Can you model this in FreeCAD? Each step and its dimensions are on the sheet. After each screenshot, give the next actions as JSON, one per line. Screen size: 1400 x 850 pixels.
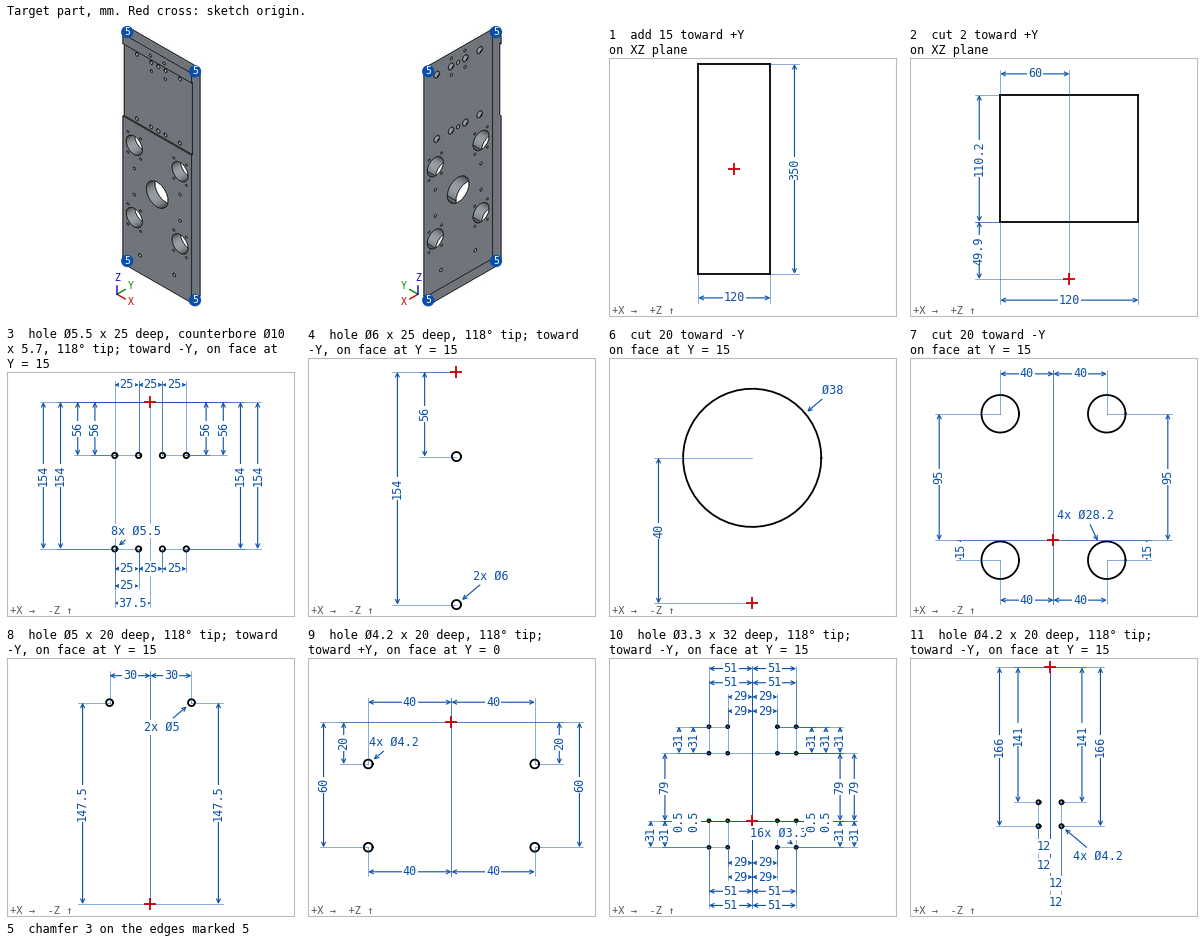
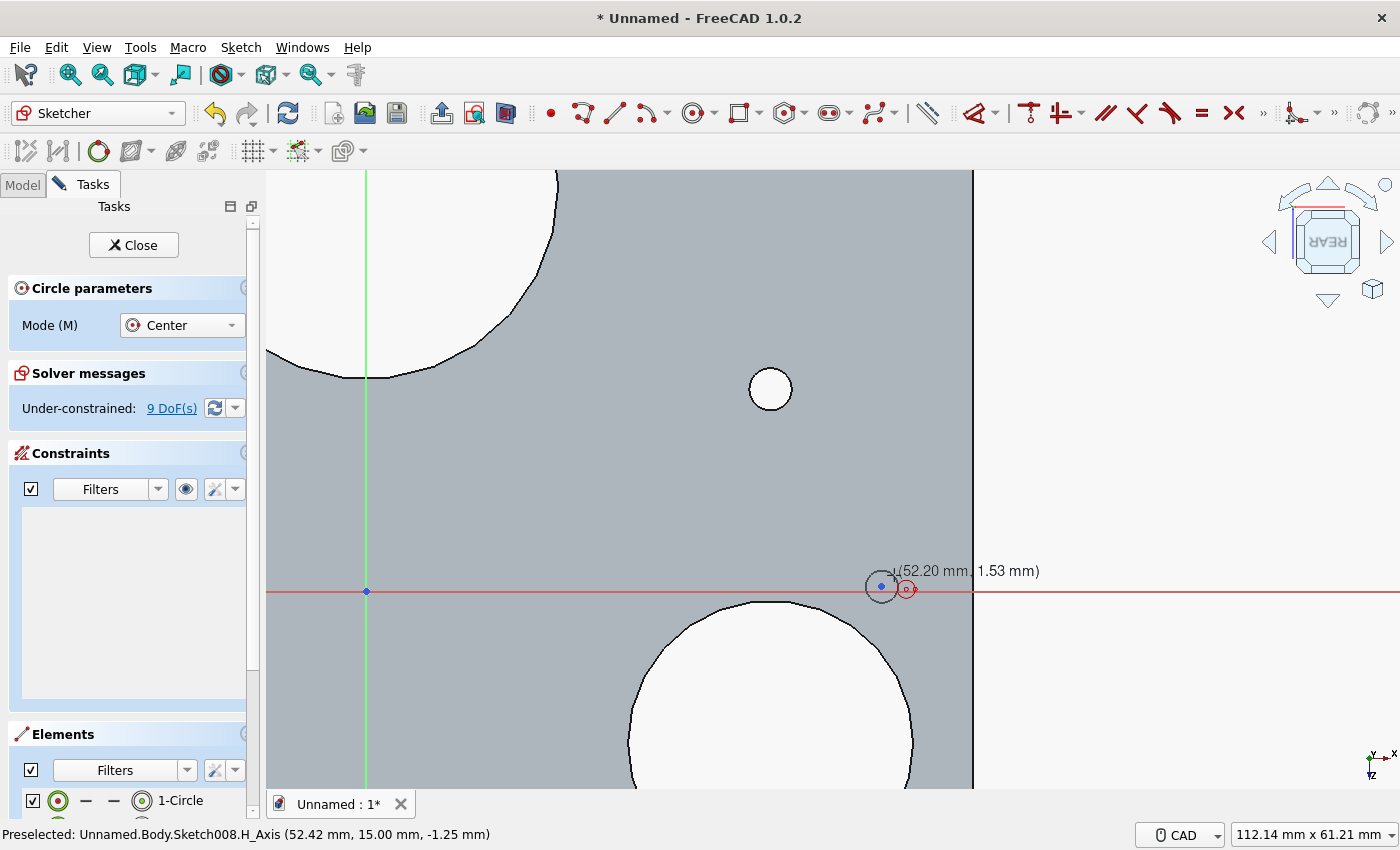
{"action": "scroll", "coordinate": [659, 586], "scroll_direction": "up", "scroll_amount": 6}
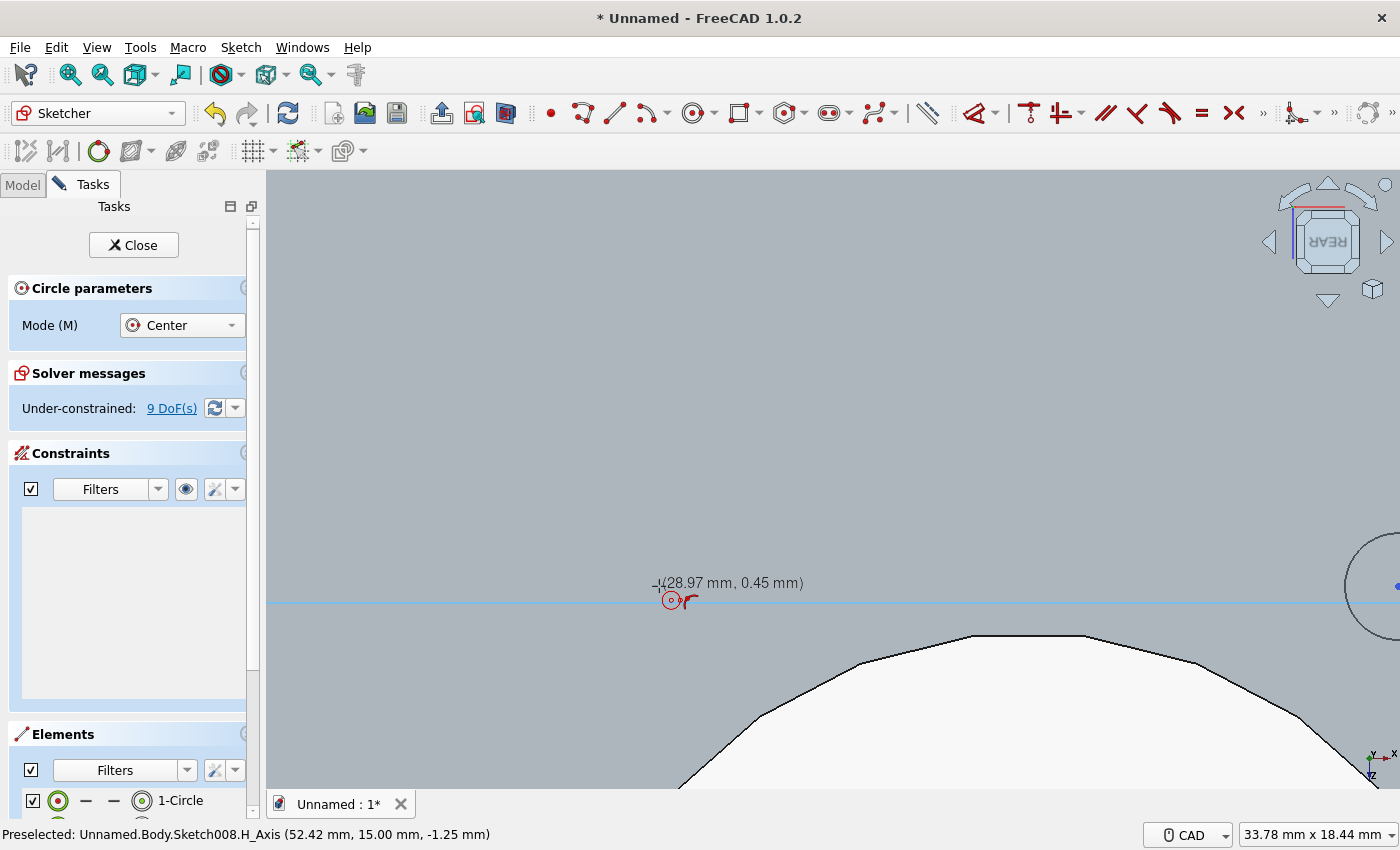
{"action": "left_click", "coordinate": [659, 586]}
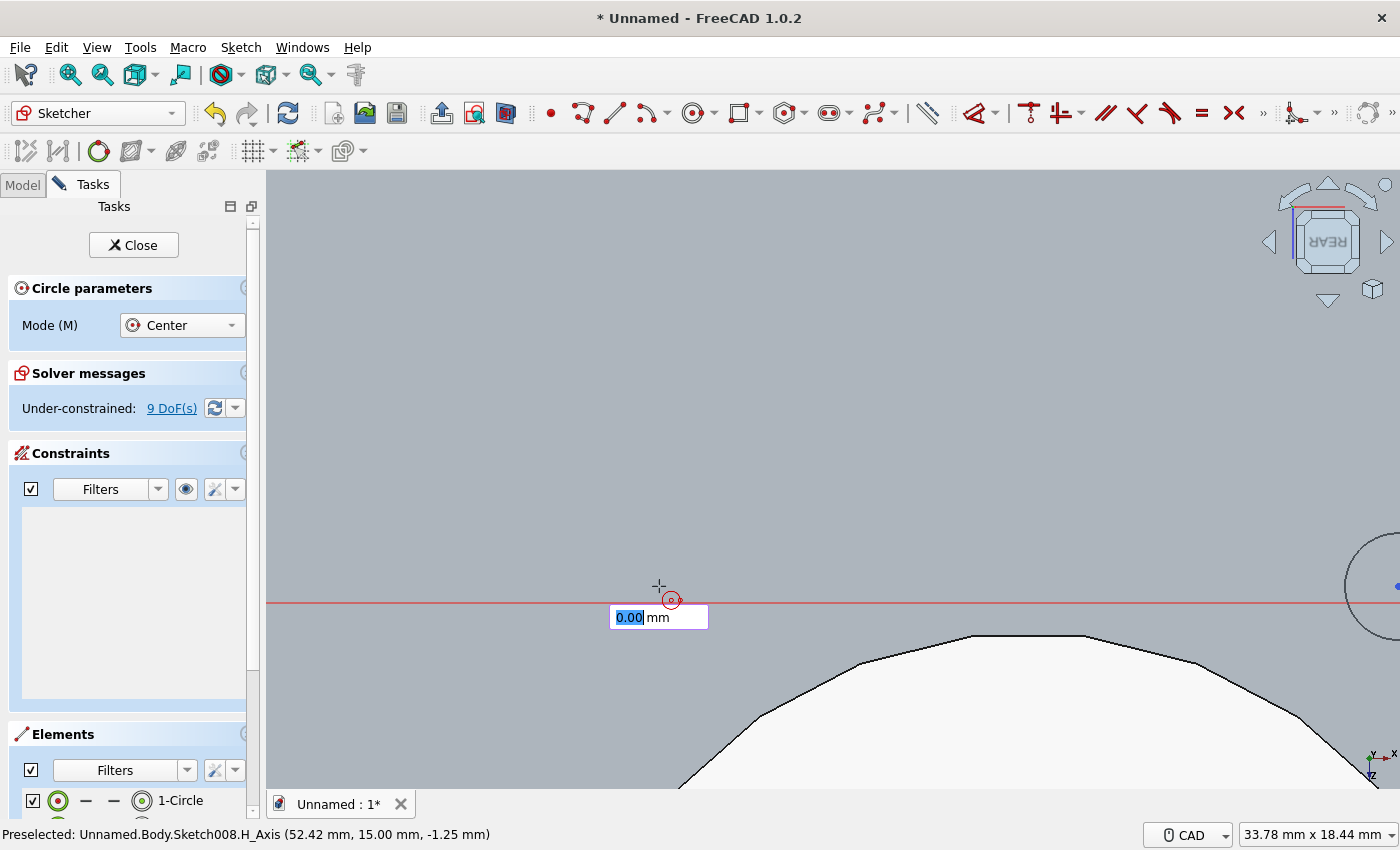
{"action": "scroll", "coordinate": [851, 577], "scroll_direction": "down", "scroll_amount": 13}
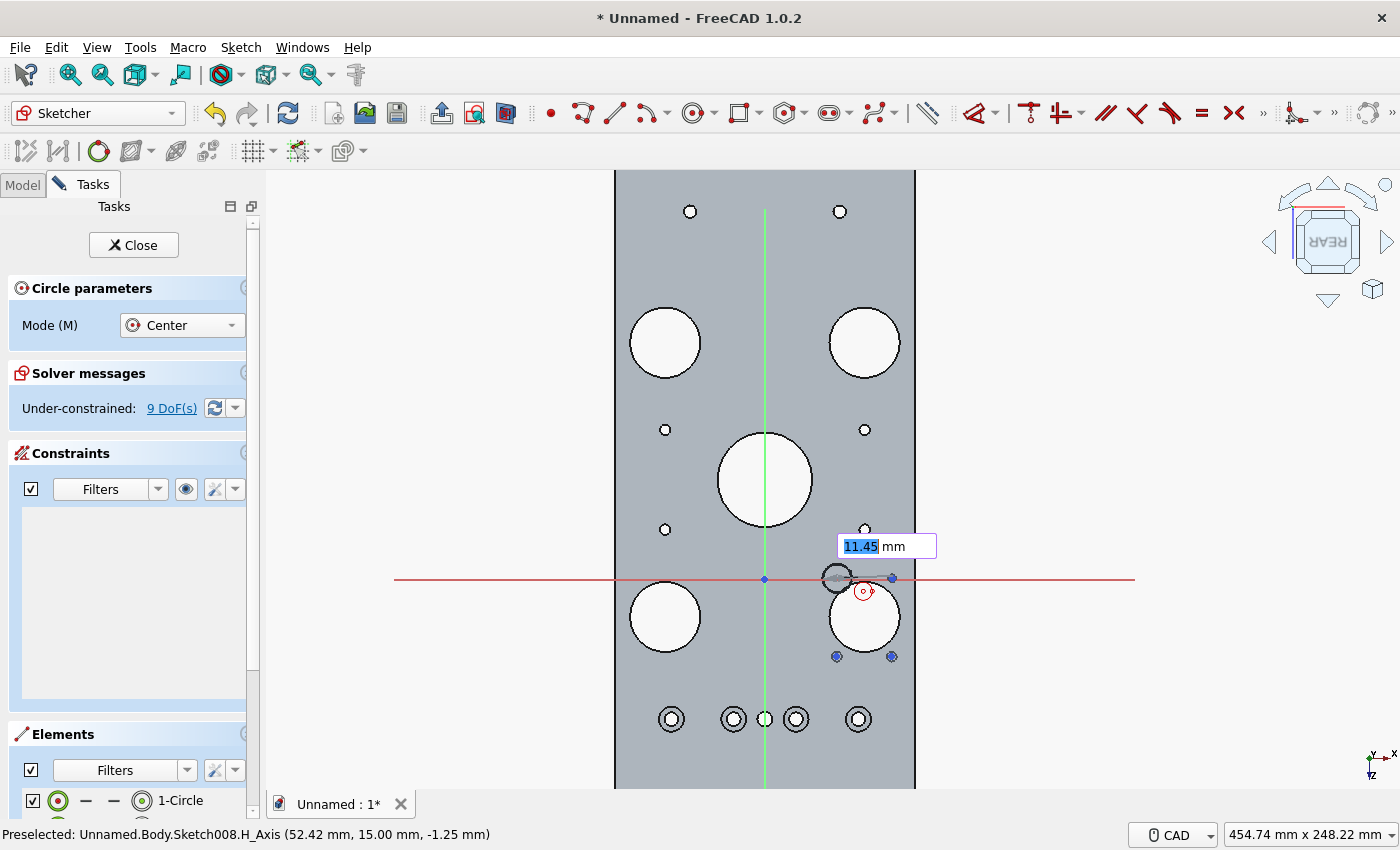
{"action": "scroll", "coordinate": [840, 575], "scroll_direction": "up", "scroll_amount": 7}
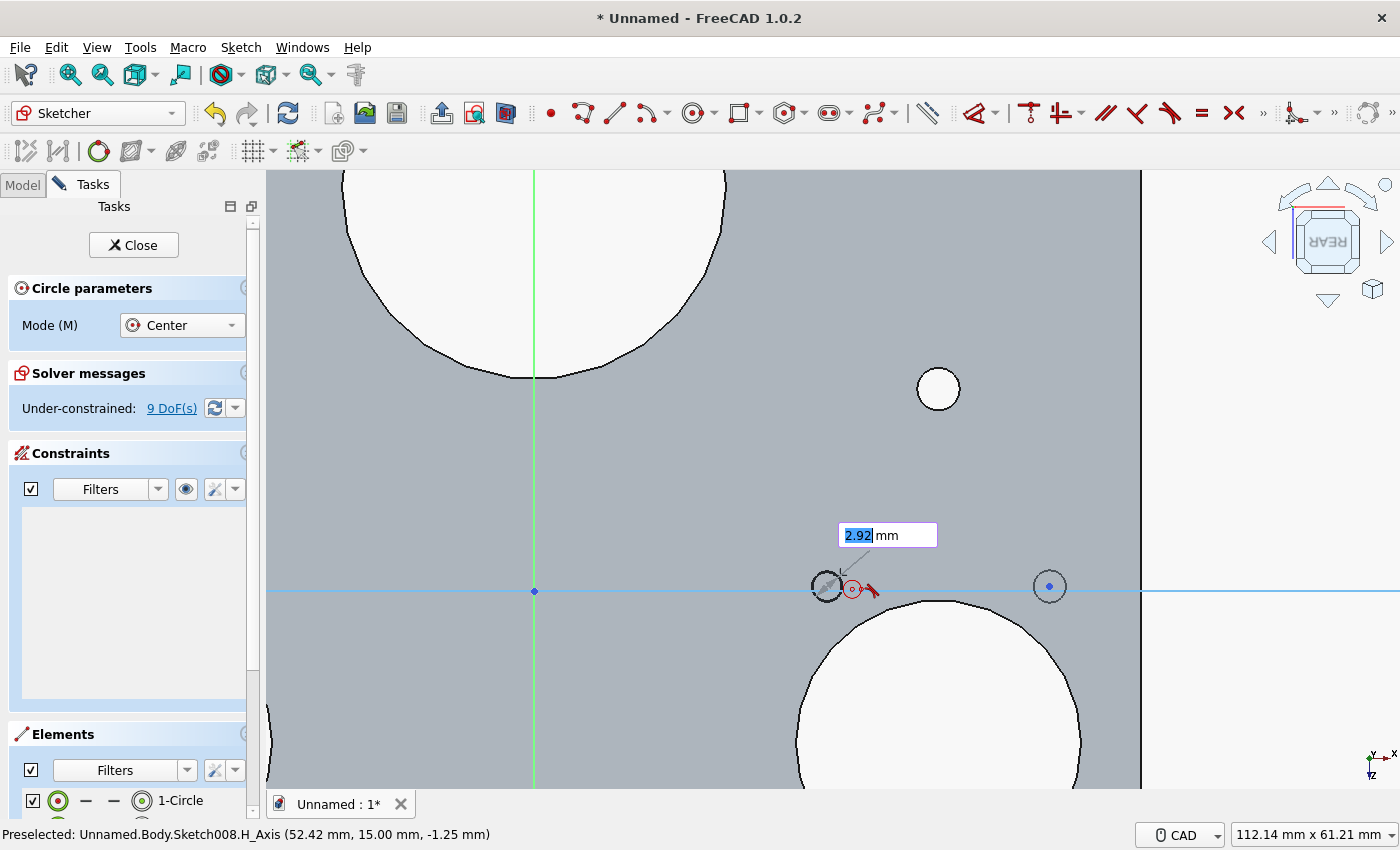
{"action": "left_click", "coordinate": [839, 574]}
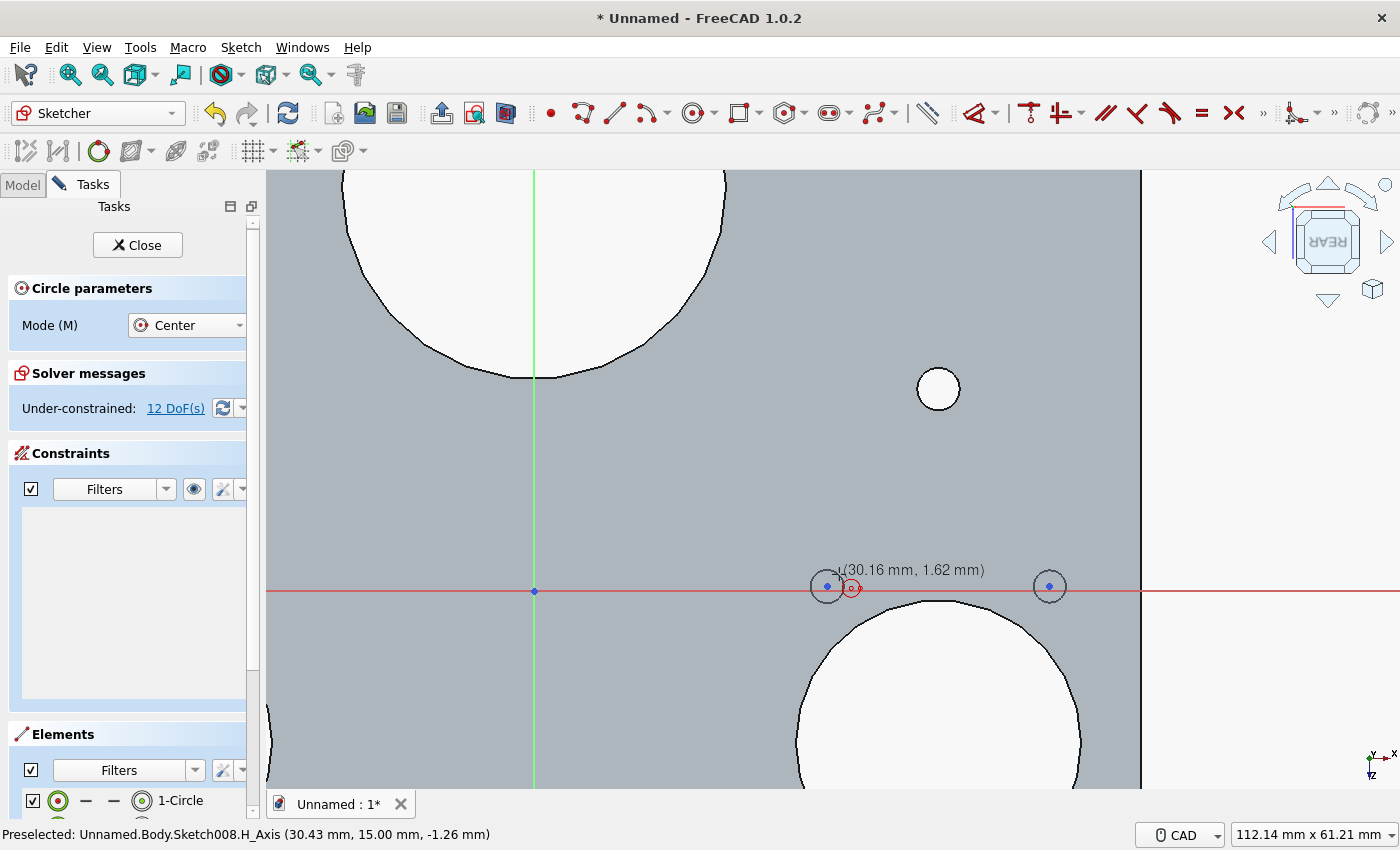
{"action": "scroll", "coordinate": [840, 575], "scroll_direction": "down", "scroll_amount": 7}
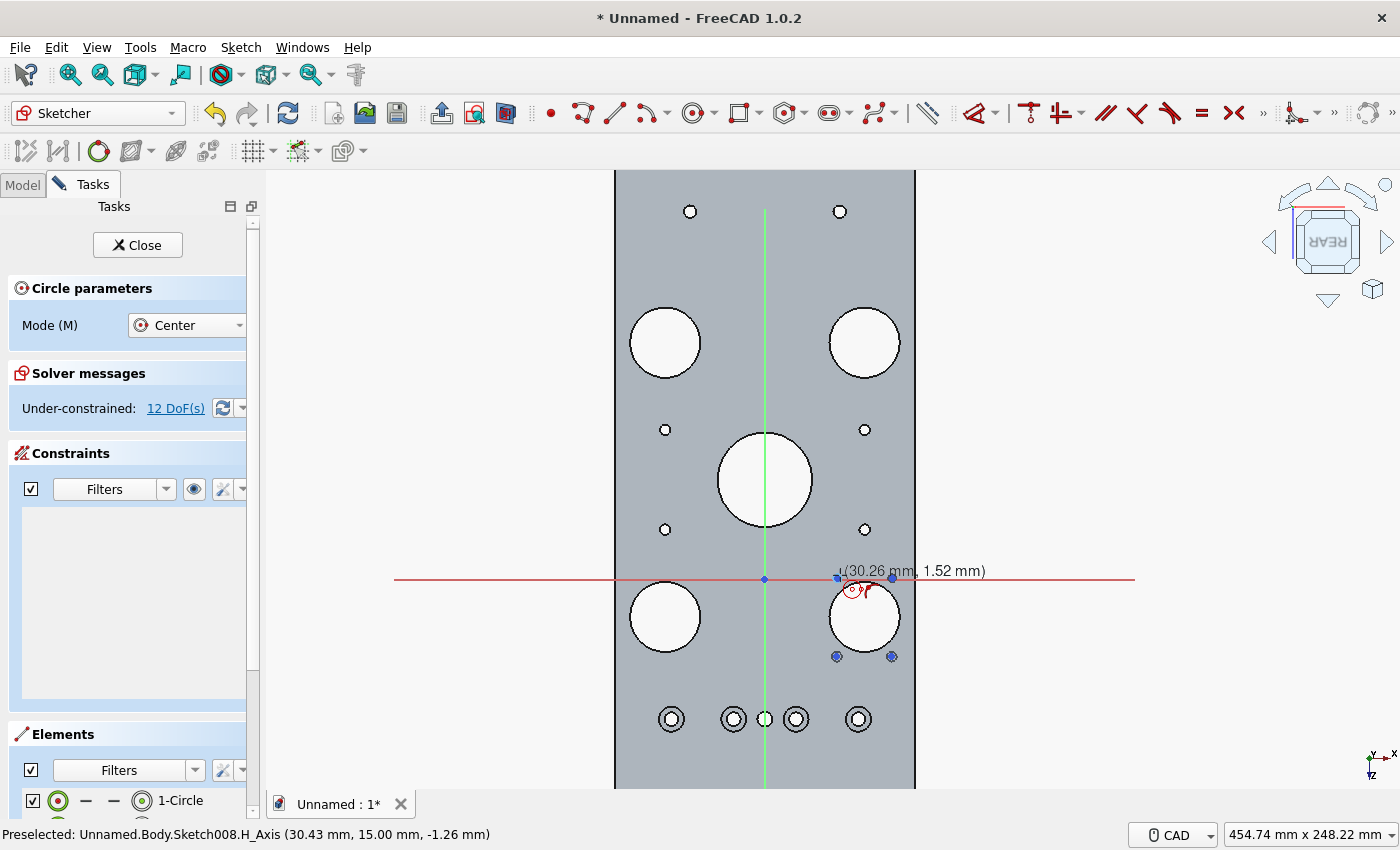
{"action": "scroll", "coordinate": [638, 656], "scroll_direction": "up", "scroll_amount": 9}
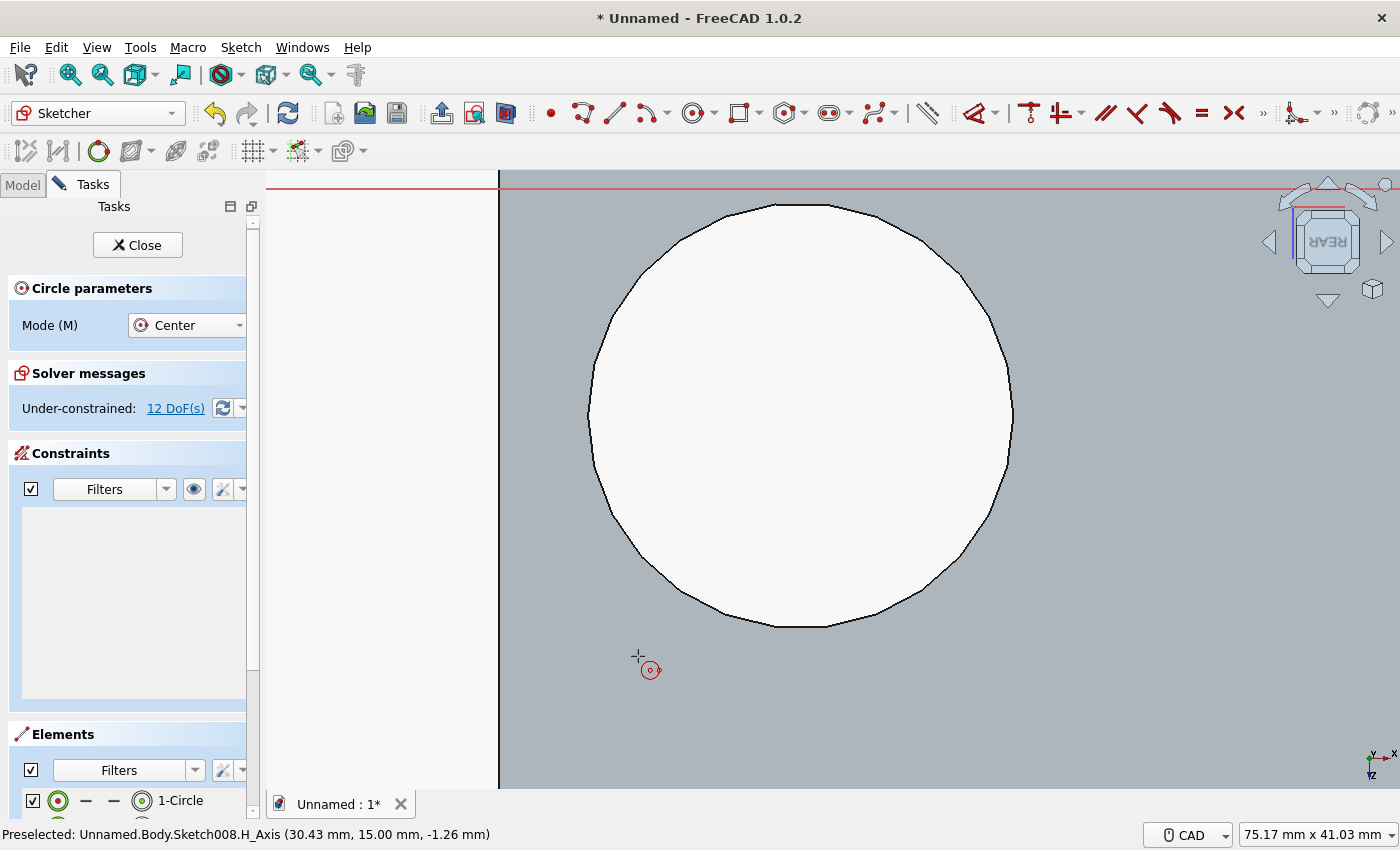
{"action": "scroll", "coordinate": [638, 656], "scroll_direction": "down", "scroll_amount": 9}